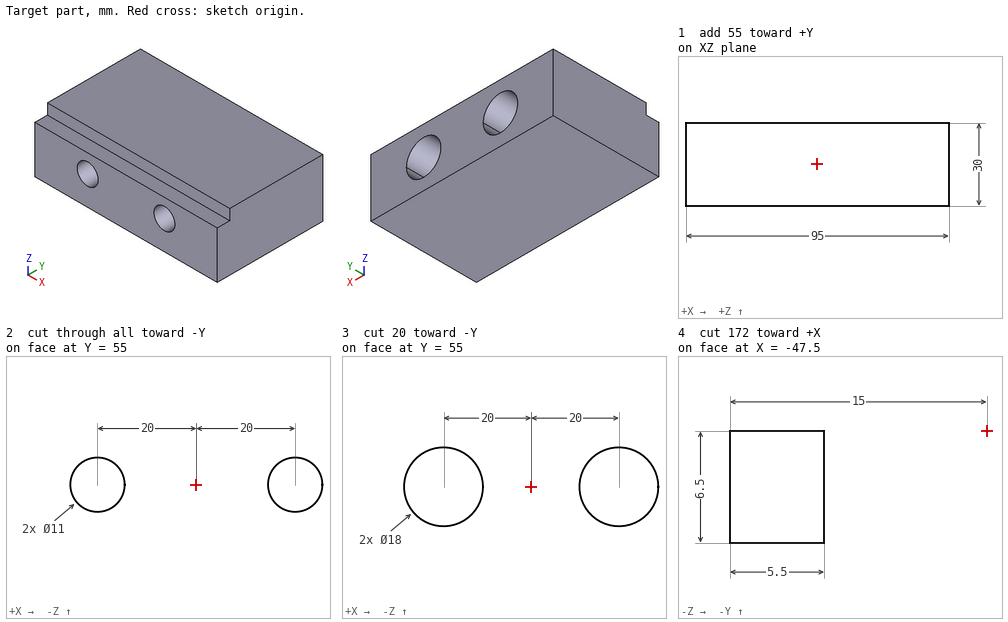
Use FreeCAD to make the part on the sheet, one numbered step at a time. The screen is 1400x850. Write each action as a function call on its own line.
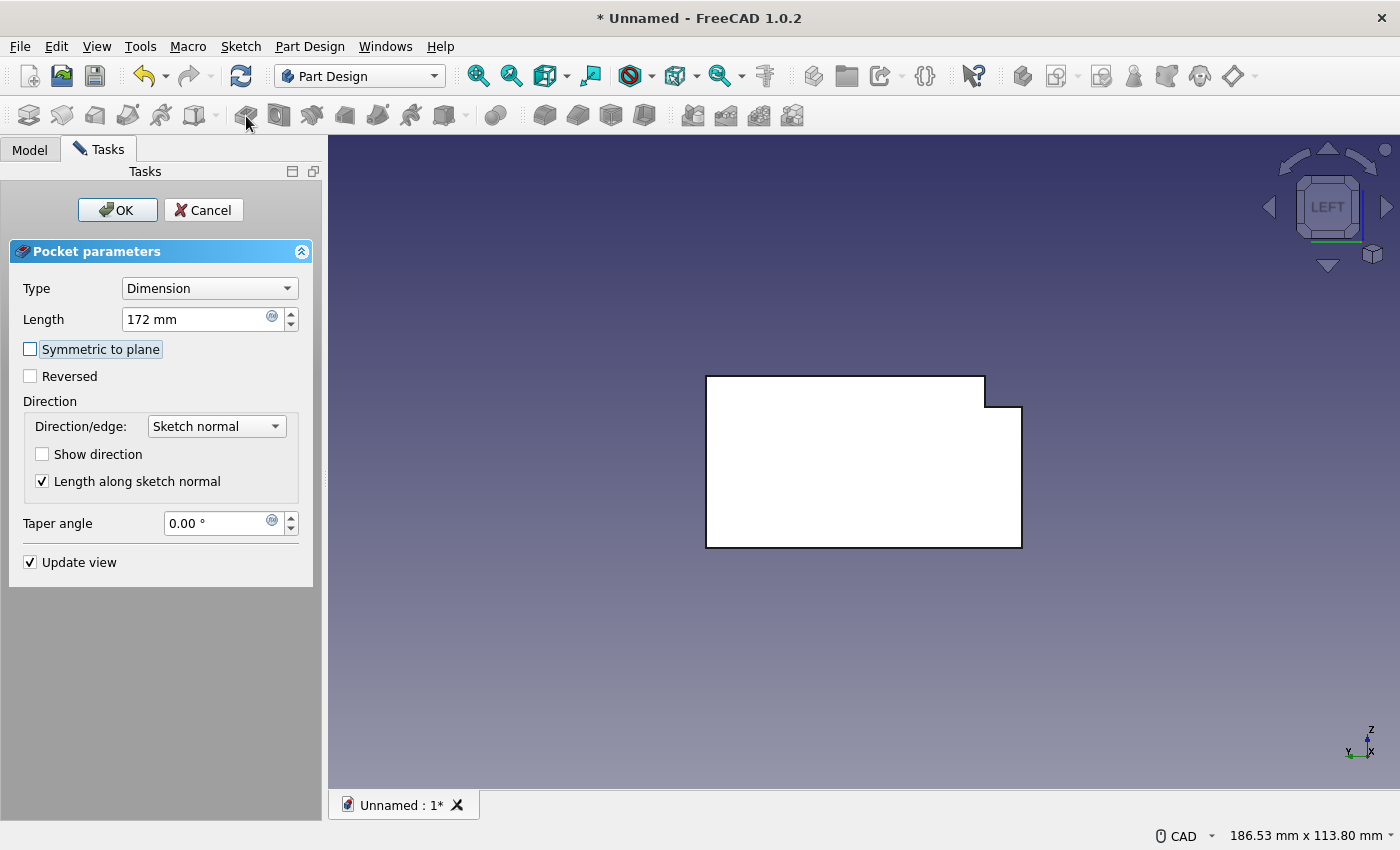
click(118, 210)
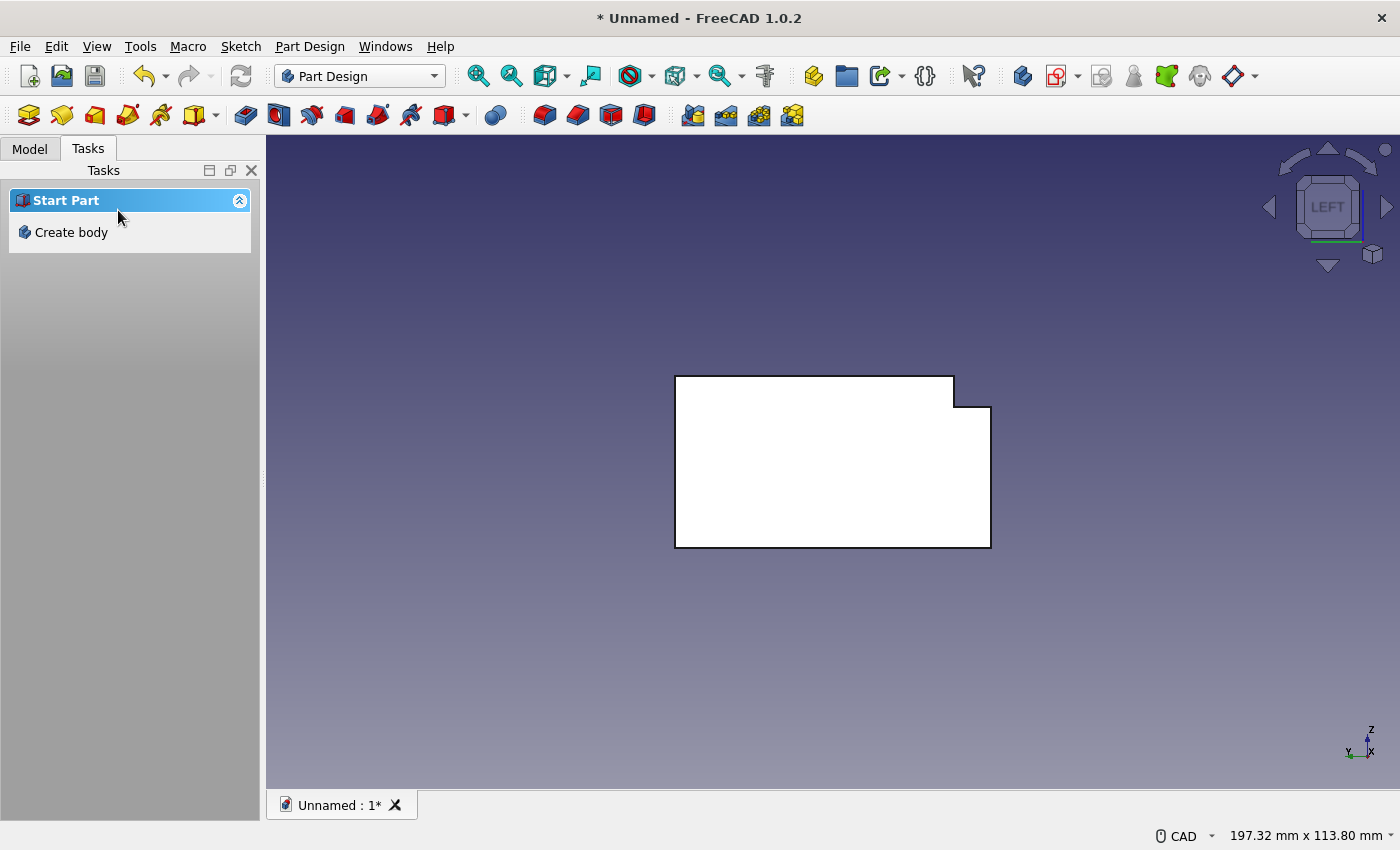
key(0)